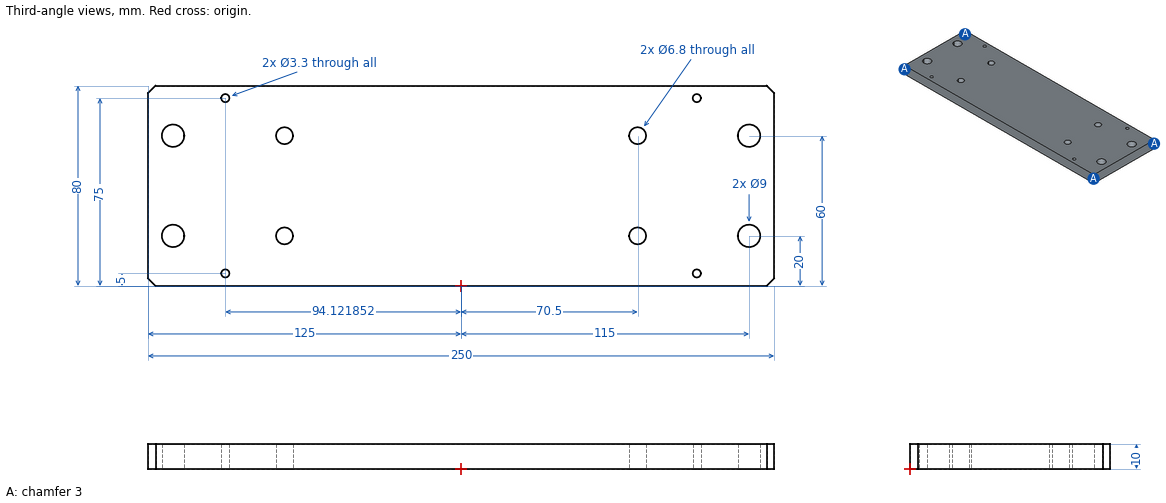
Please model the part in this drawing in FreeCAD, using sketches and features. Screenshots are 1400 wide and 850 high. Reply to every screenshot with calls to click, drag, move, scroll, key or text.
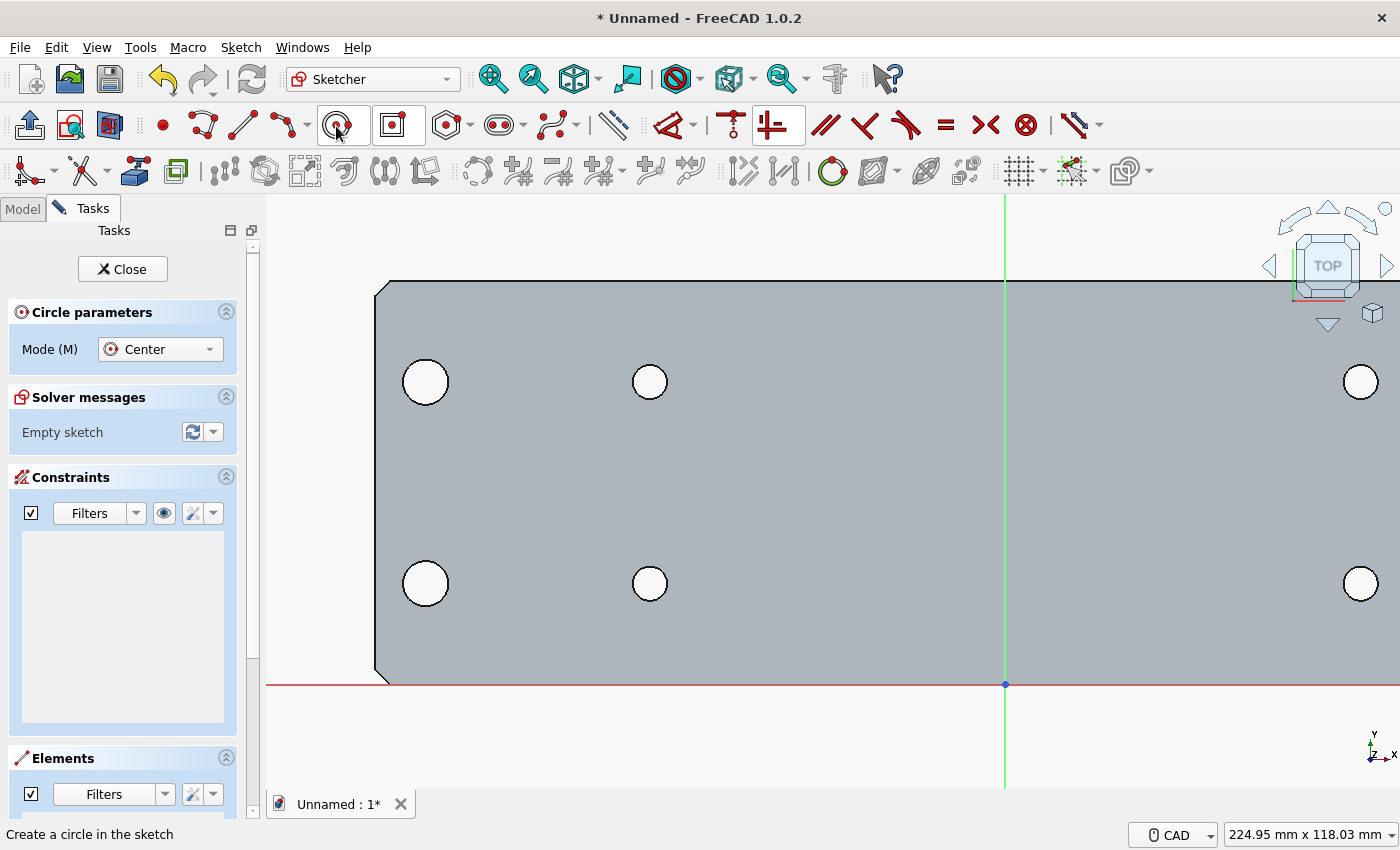
scroll(531, 306, up, 6)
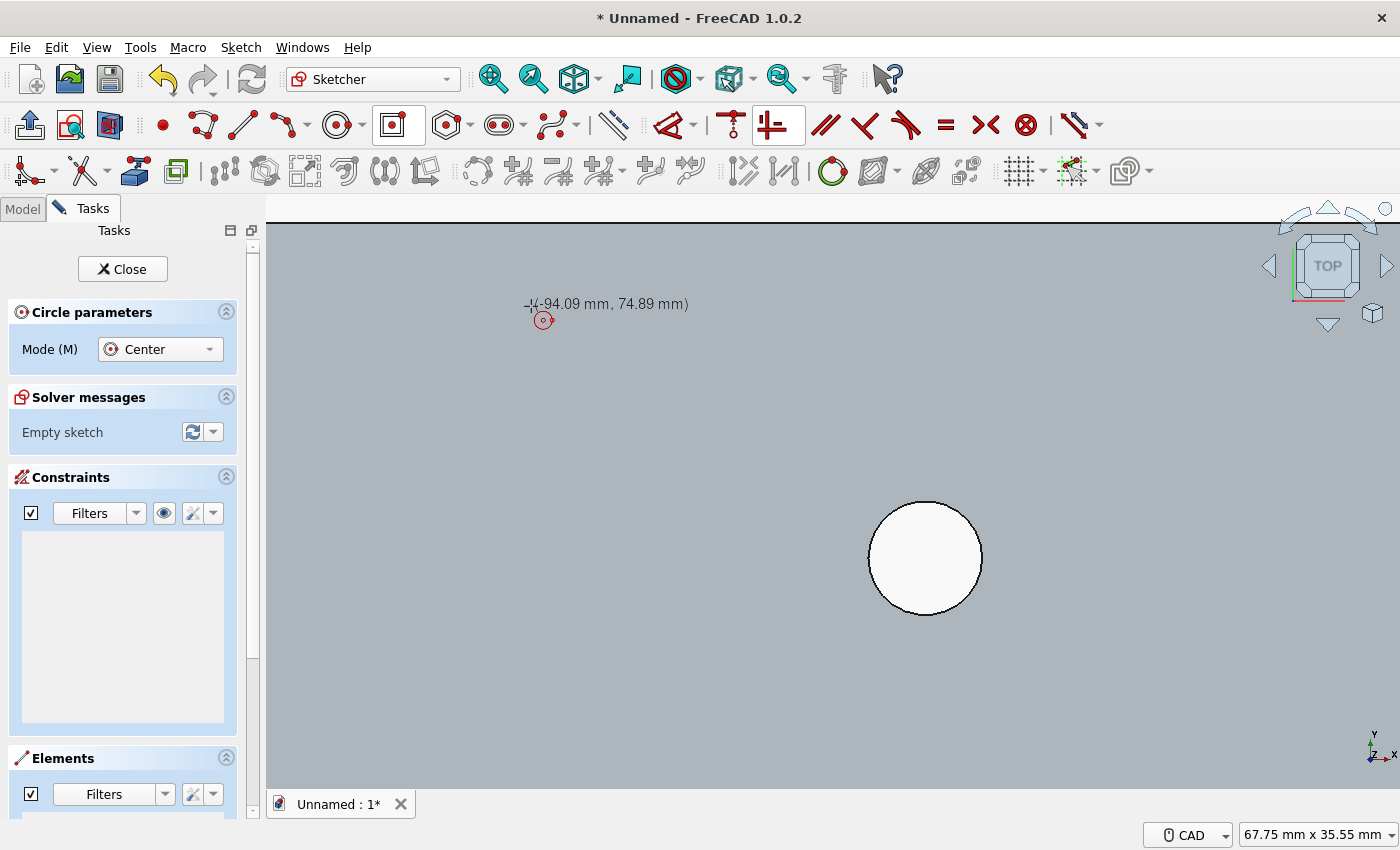
click(530, 307)
move(550, 288)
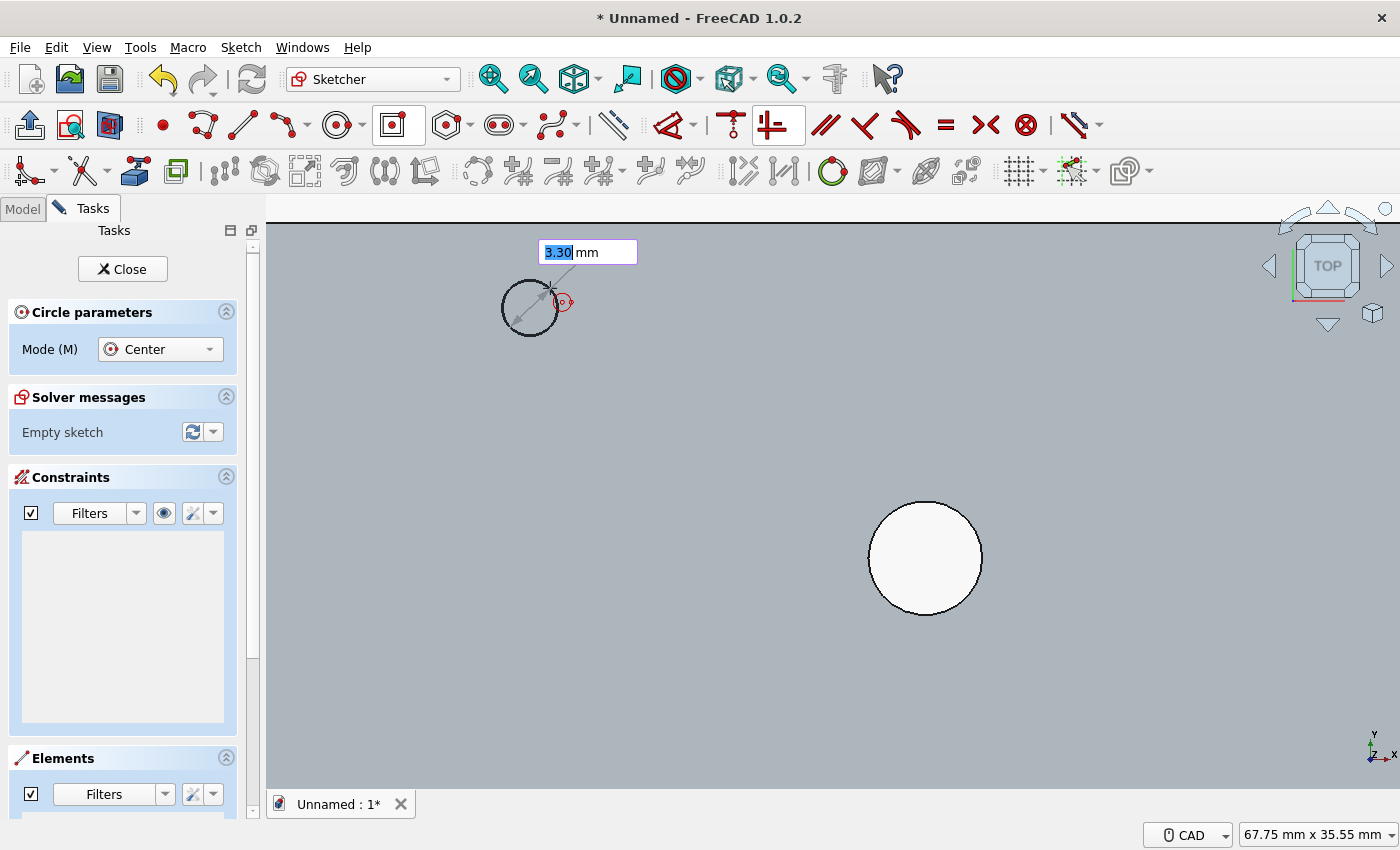
text(3.3)
key(Return)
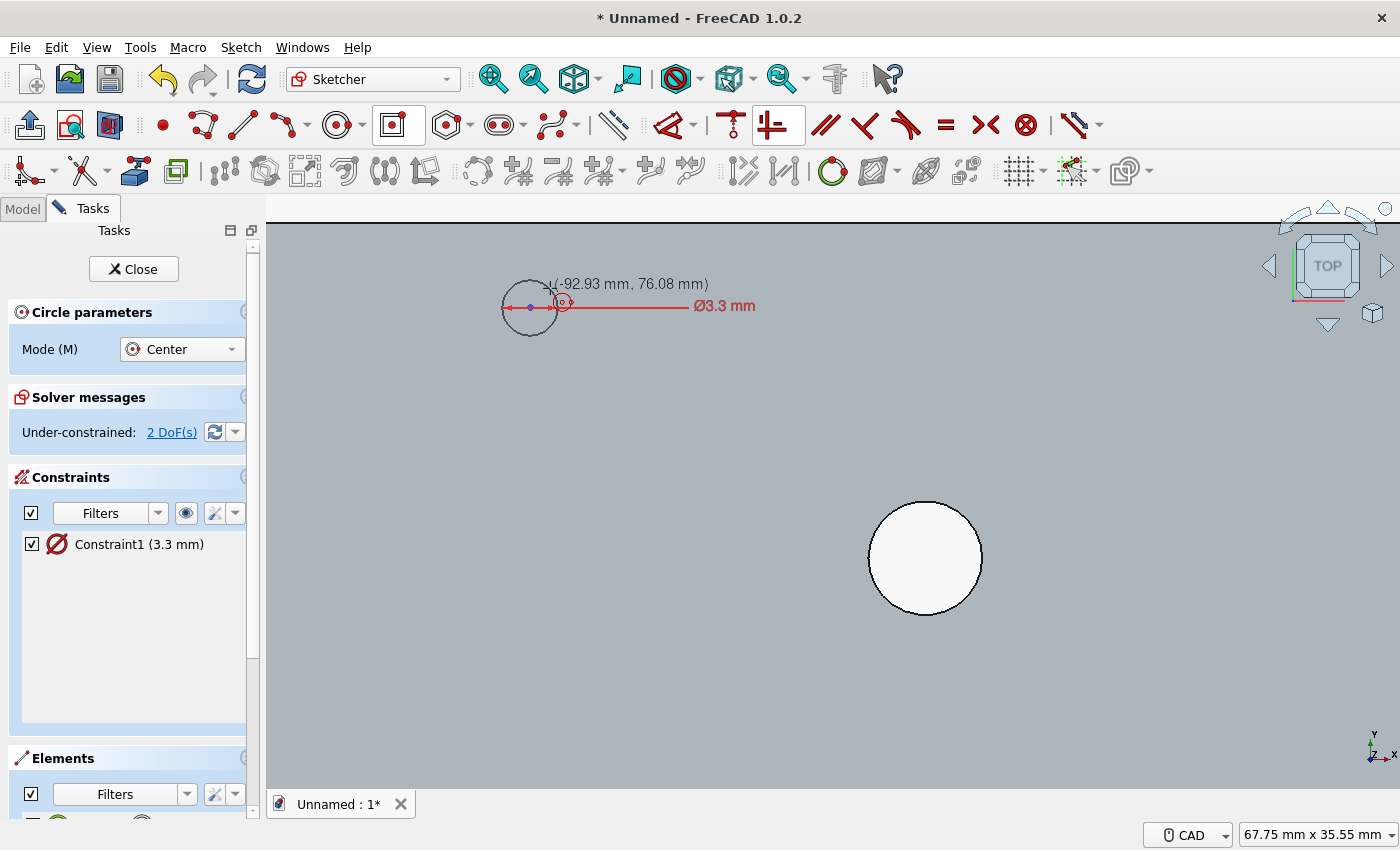
scroll(532, 306, down, 6)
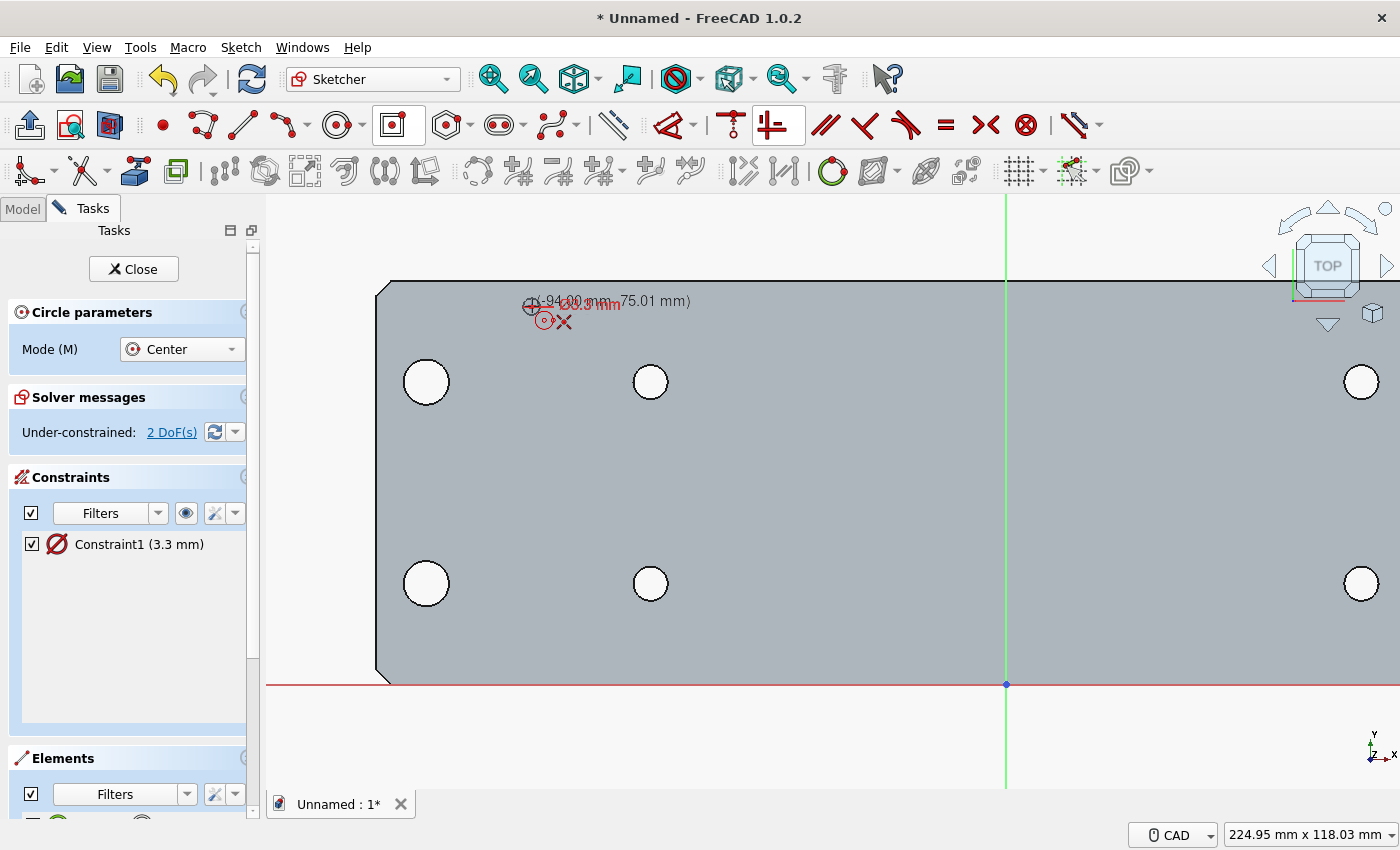
scroll(532, 659, up, 6)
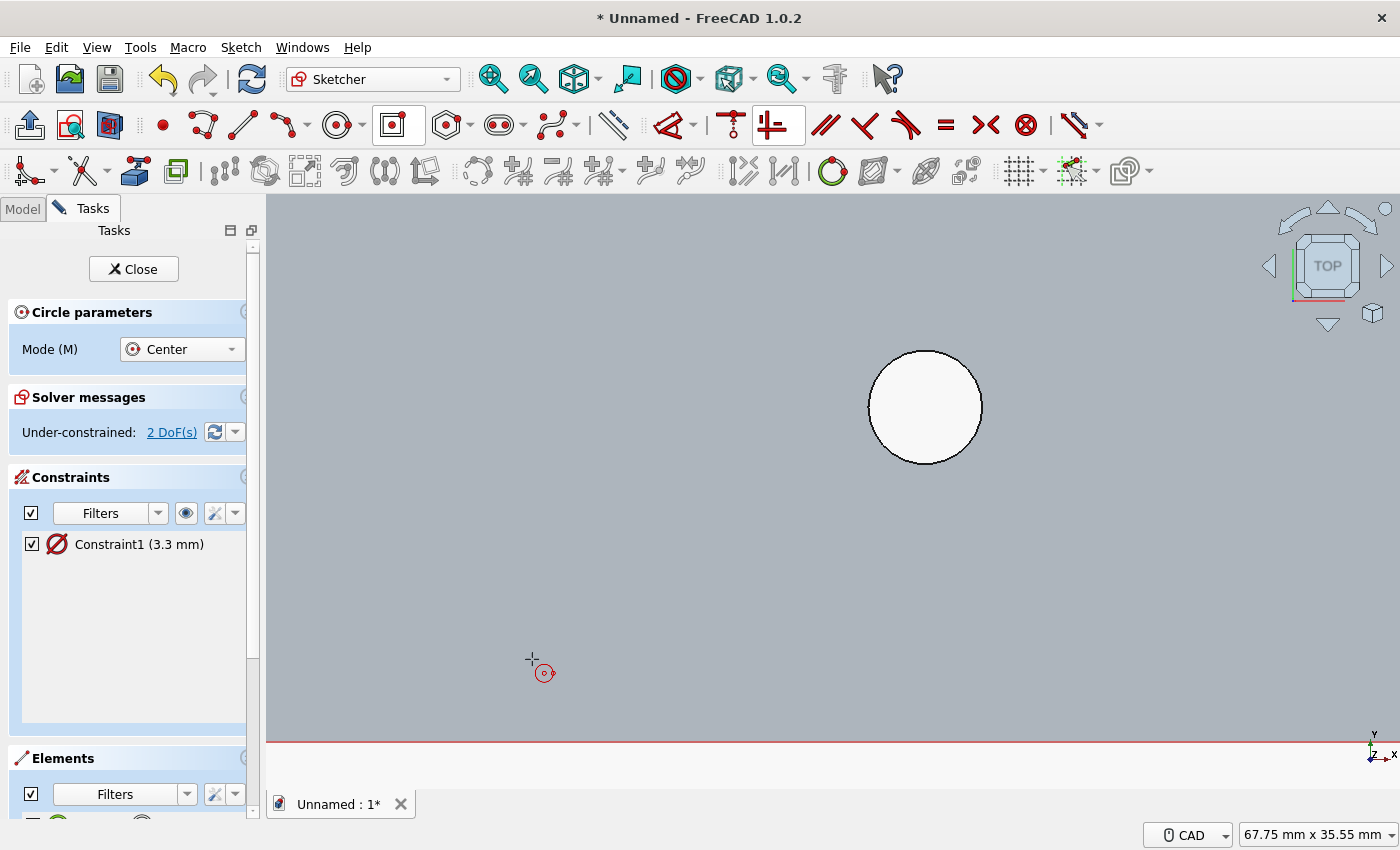
click(530, 658)
move(550, 639)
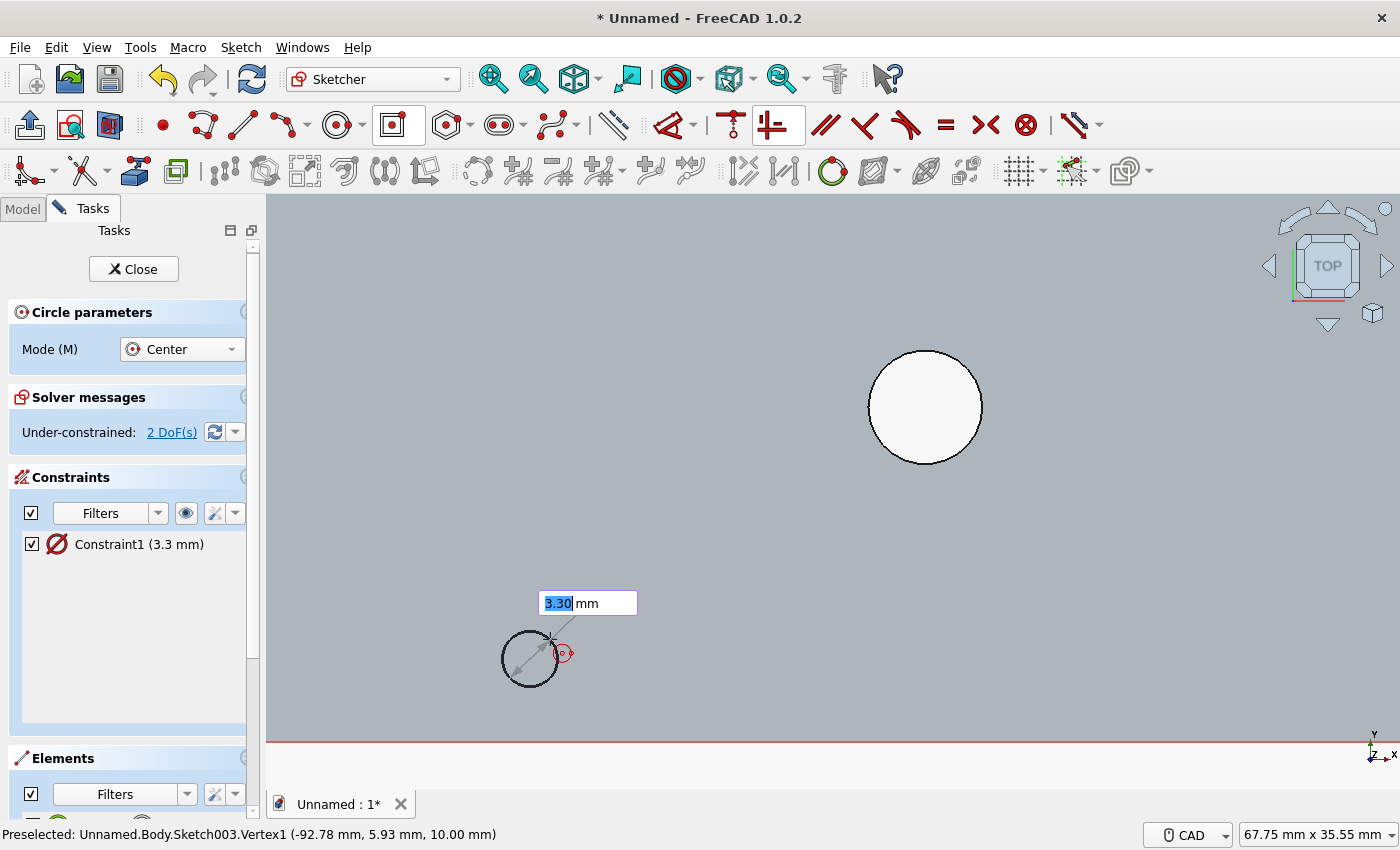
text(3.3)
key(Return)
key(Escape)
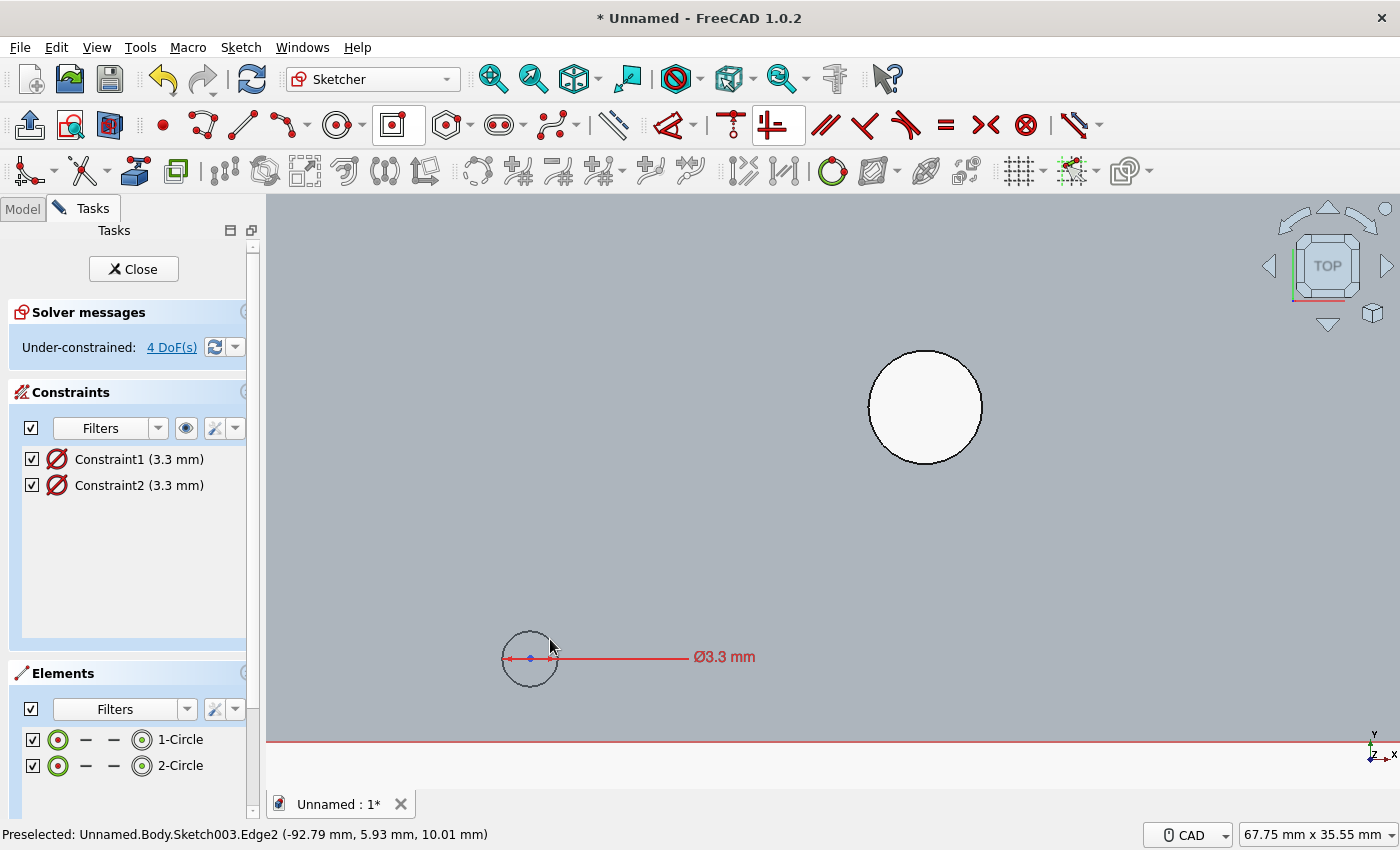
scroll(532, 660, down, 6)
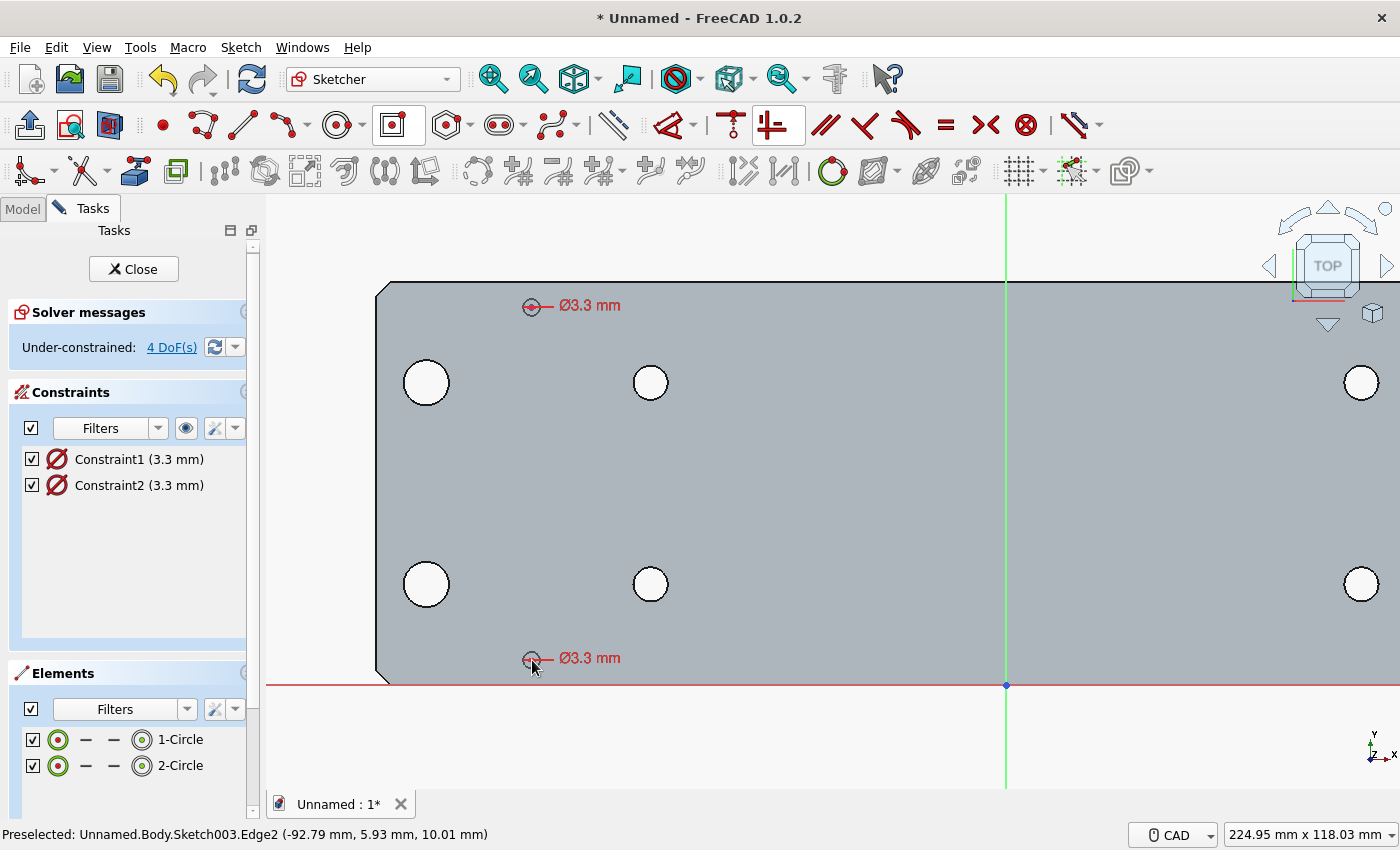
click(532, 307)